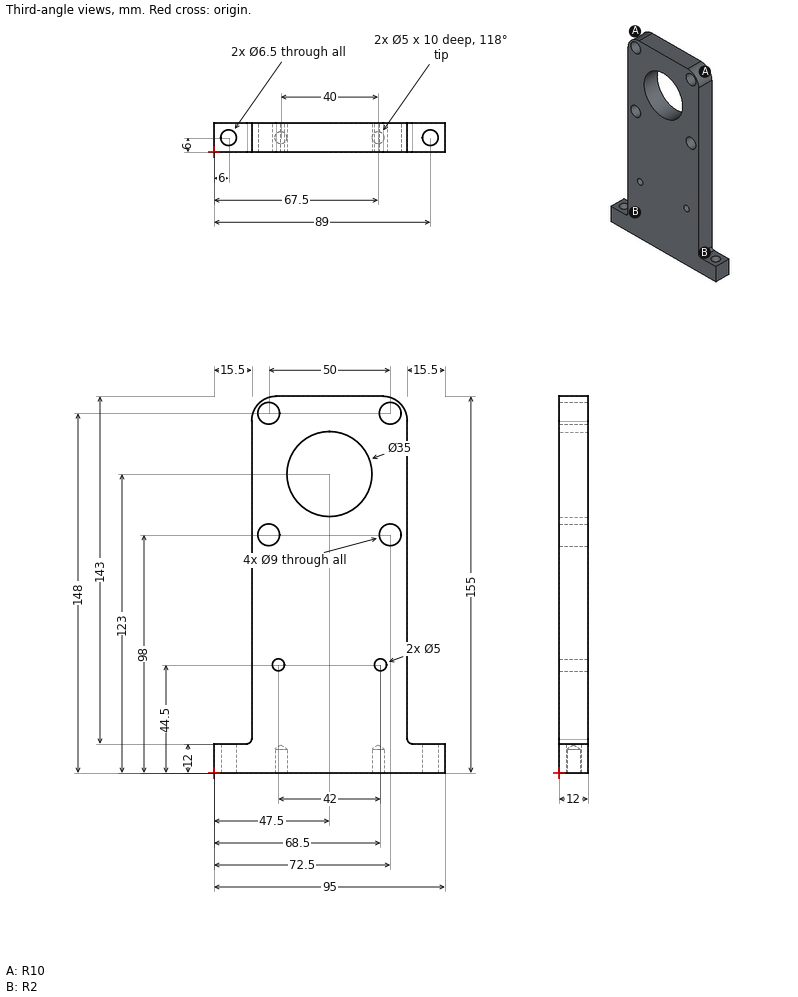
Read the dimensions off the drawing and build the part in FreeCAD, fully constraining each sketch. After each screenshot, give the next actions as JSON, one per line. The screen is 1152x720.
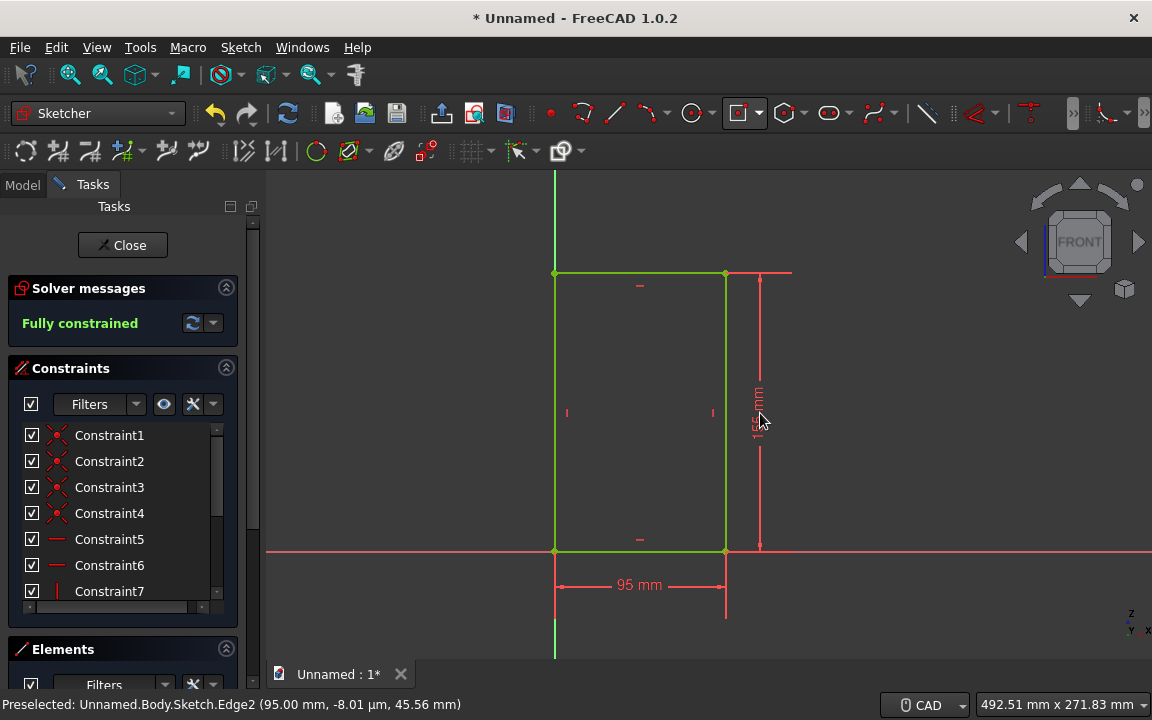
{"action": "left_click", "coordinate": [123, 245]}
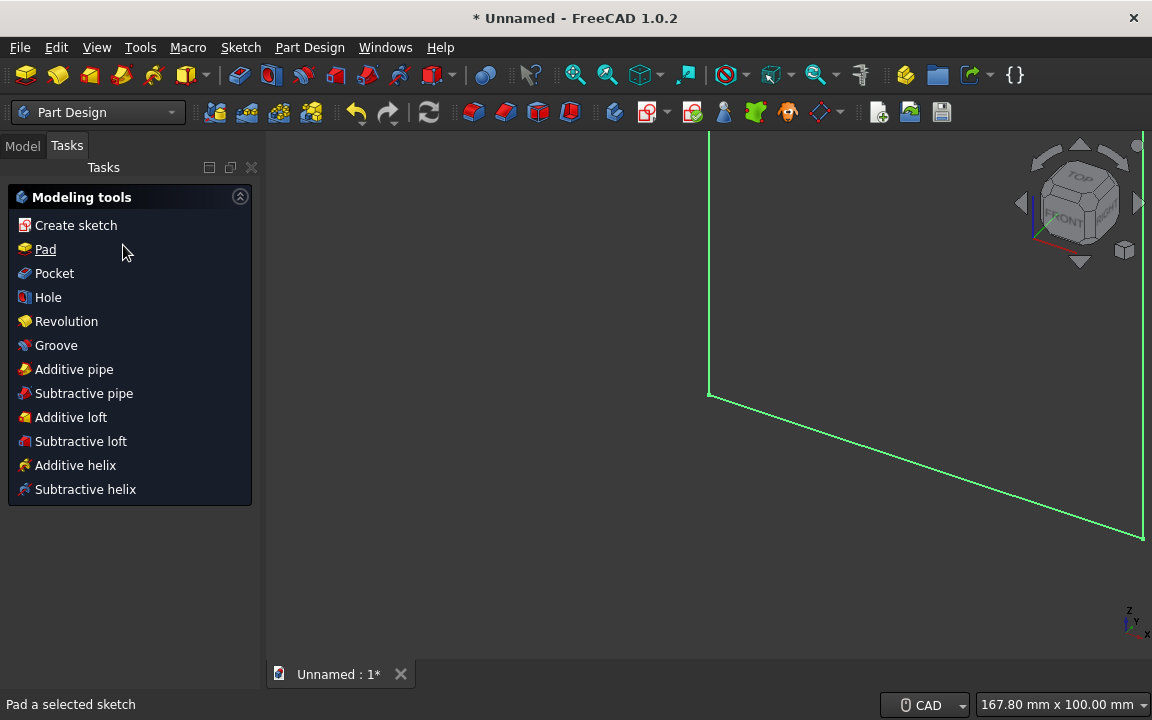
{"action": "left_click", "coordinate": [26, 76]}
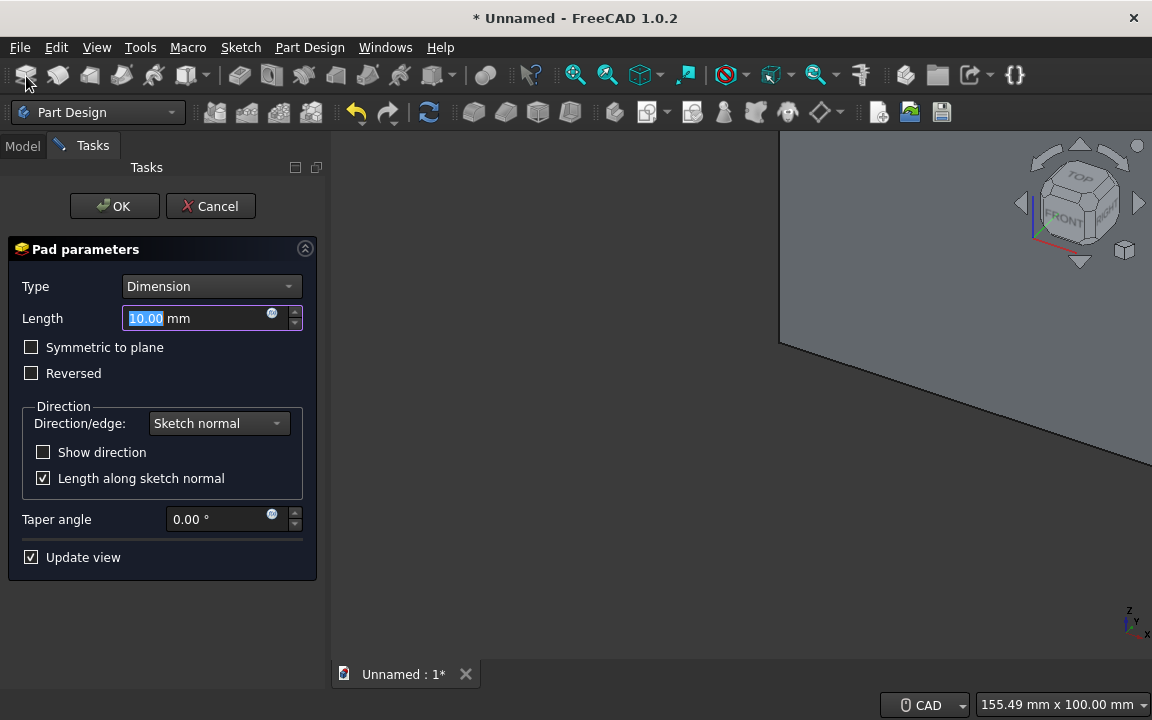
{"action": "type", "text": "12"}
{"action": "key", "text": "Tab"}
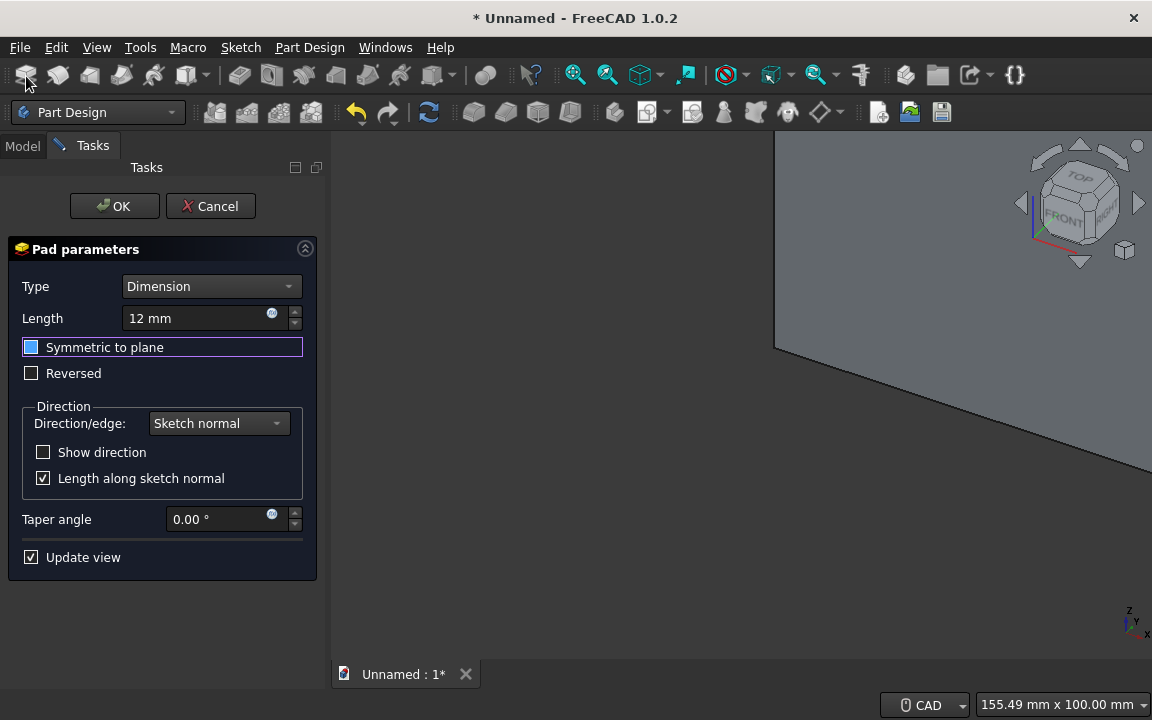
{"action": "left_click", "coordinate": [30, 373]}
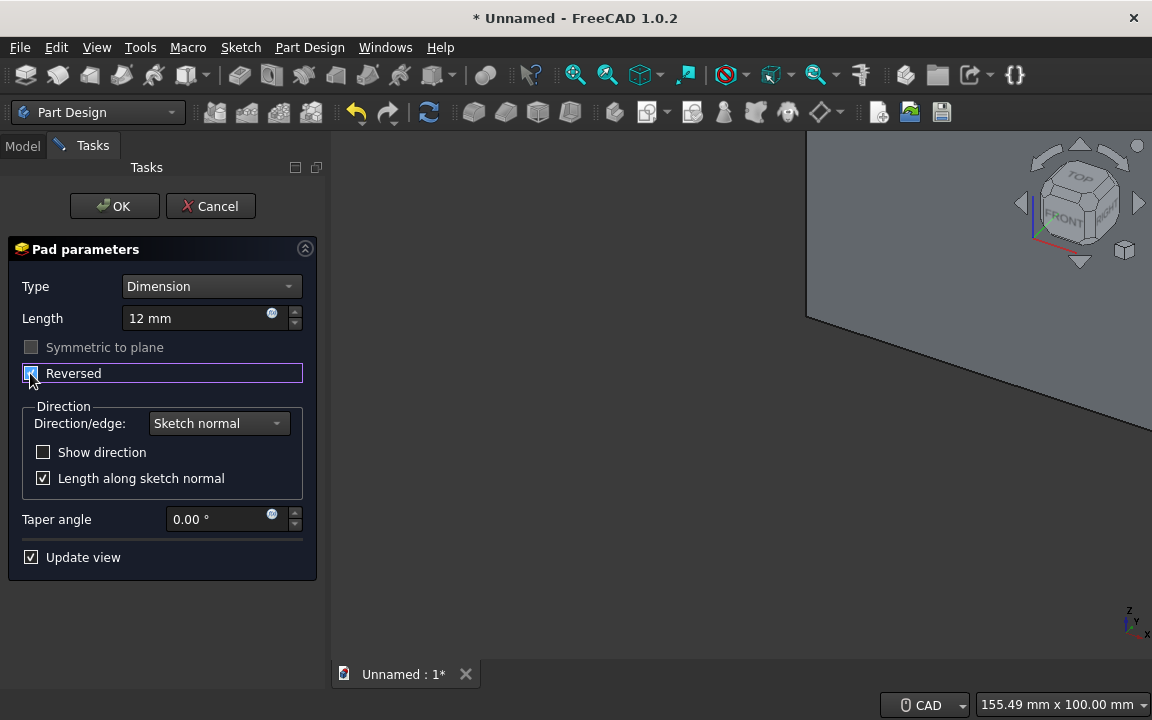
{"action": "left_click", "coordinate": [115, 206]}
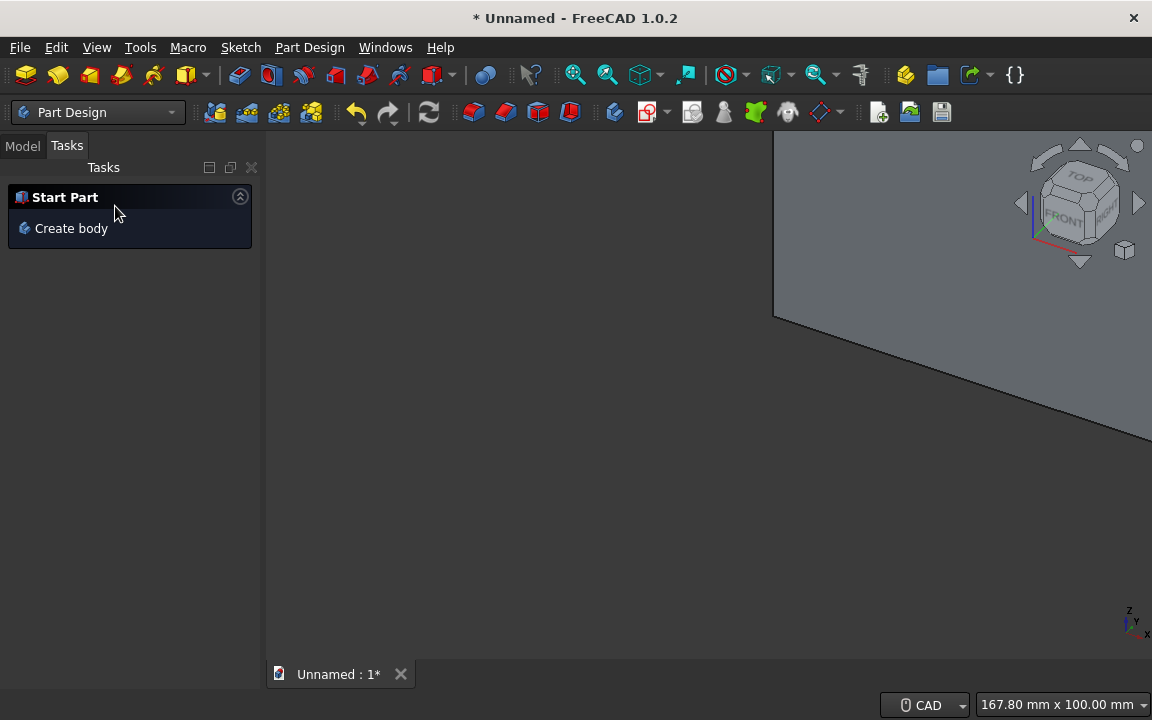
{"action": "left_click", "coordinate": [576, 76]}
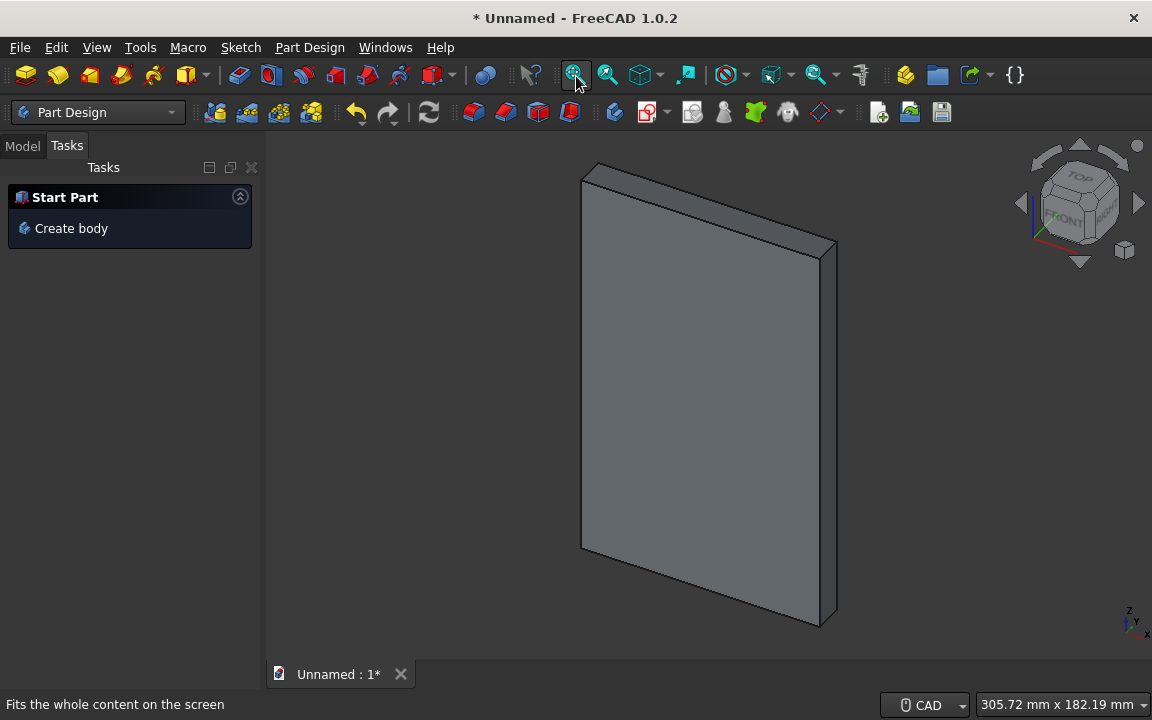
{"action": "key", "text": "4"}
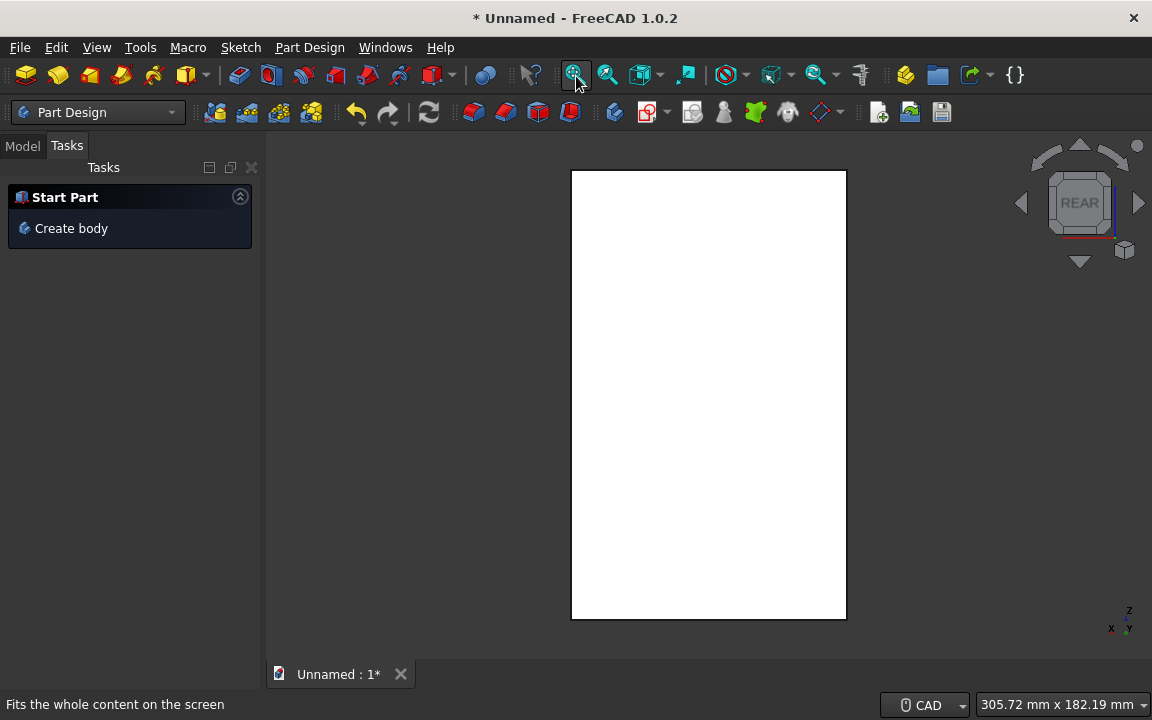
{"action": "left_click", "coordinate": [709, 330]}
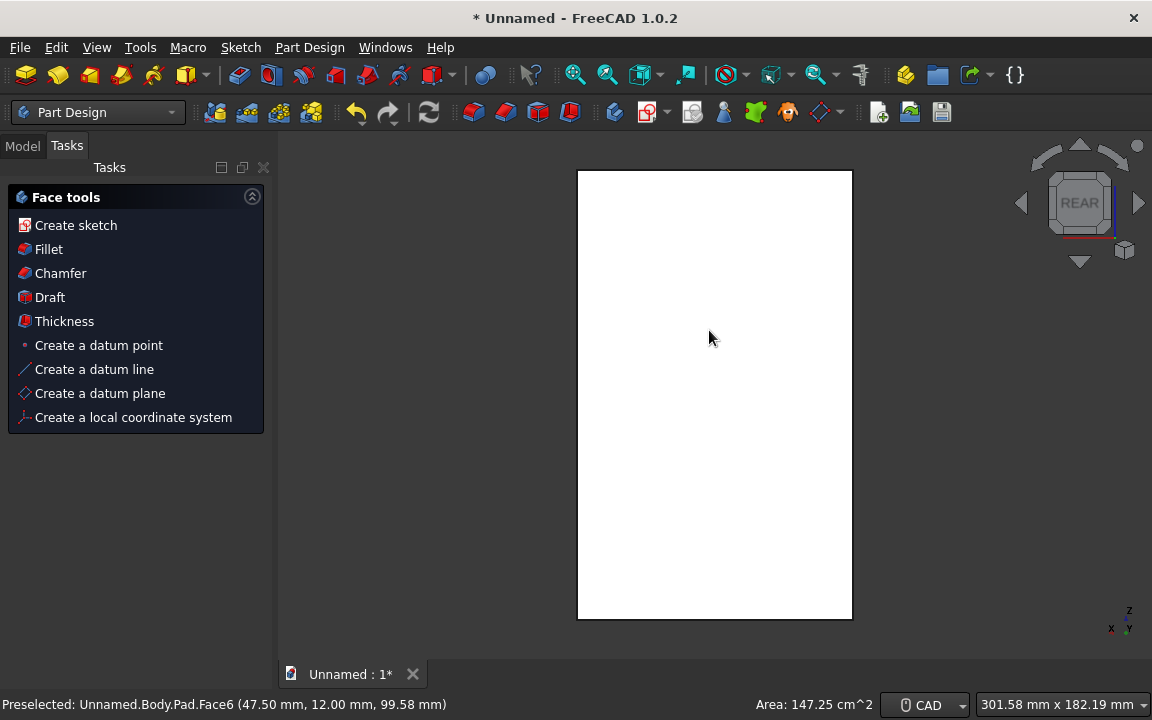
{"action": "left_click", "coordinate": [648, 112]}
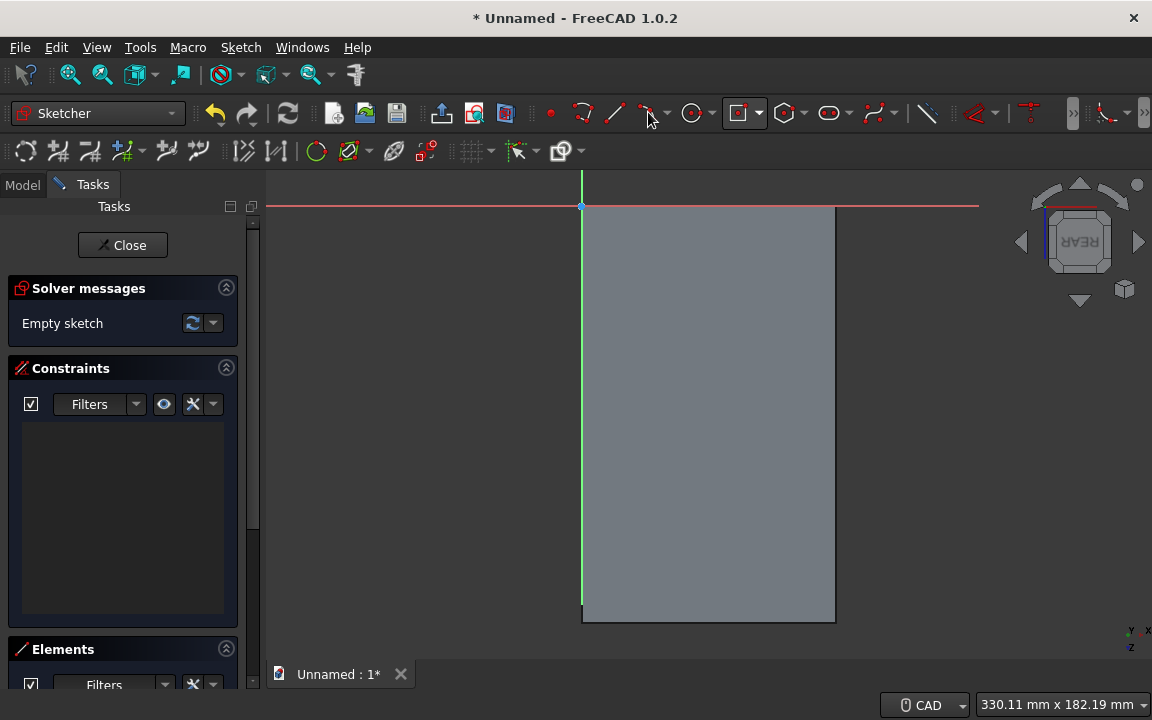
{"action": "scroll", "coordinate": [501, 415], "scroll_direction": "down", "scroll_amount": 2}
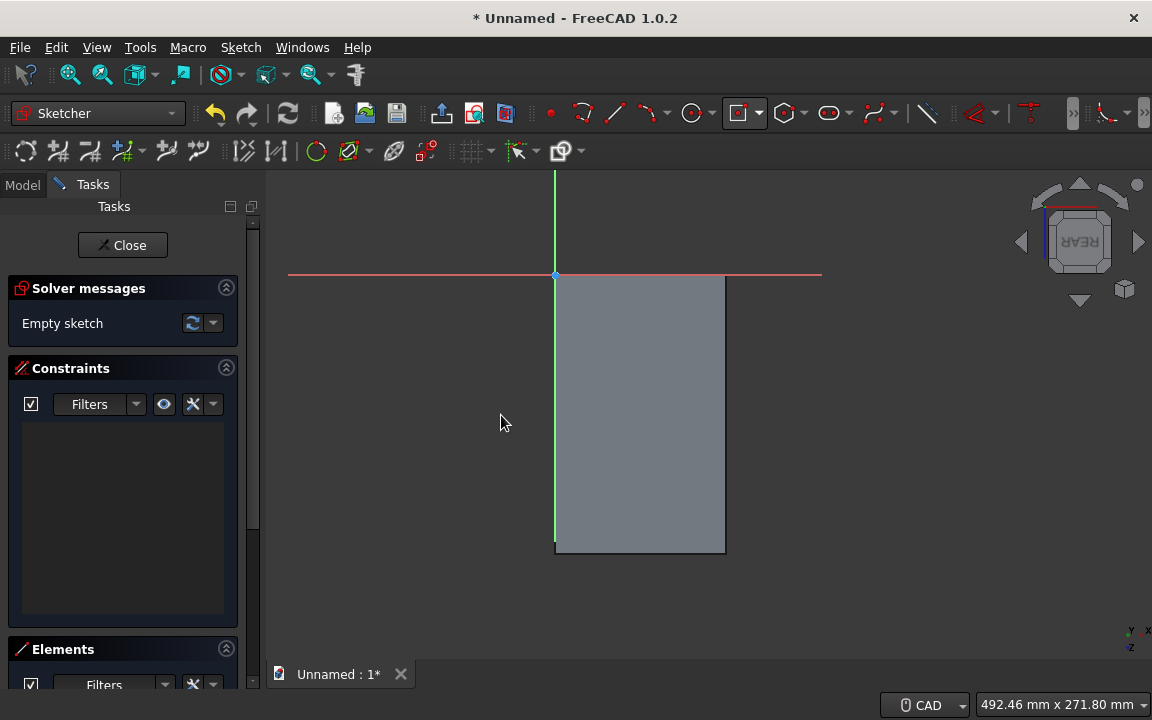
{"action": "left_click", "coordinate": [762, 114]}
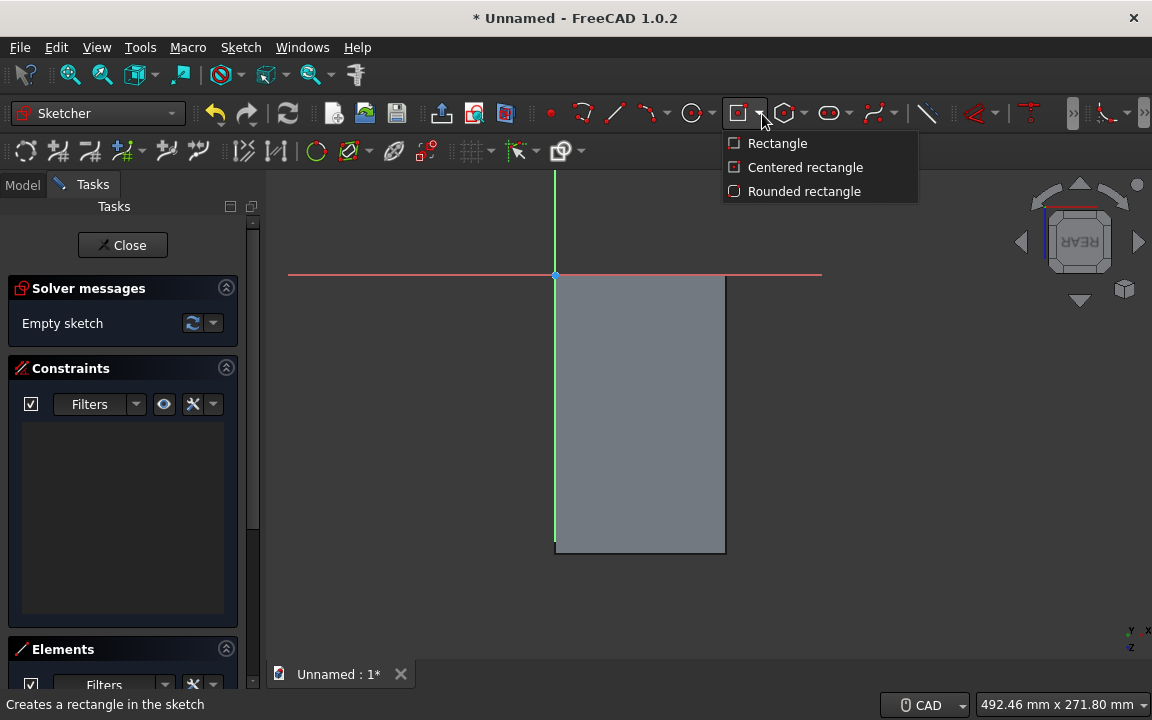
{"action": "left_click", "coordinate": [820, 143]}